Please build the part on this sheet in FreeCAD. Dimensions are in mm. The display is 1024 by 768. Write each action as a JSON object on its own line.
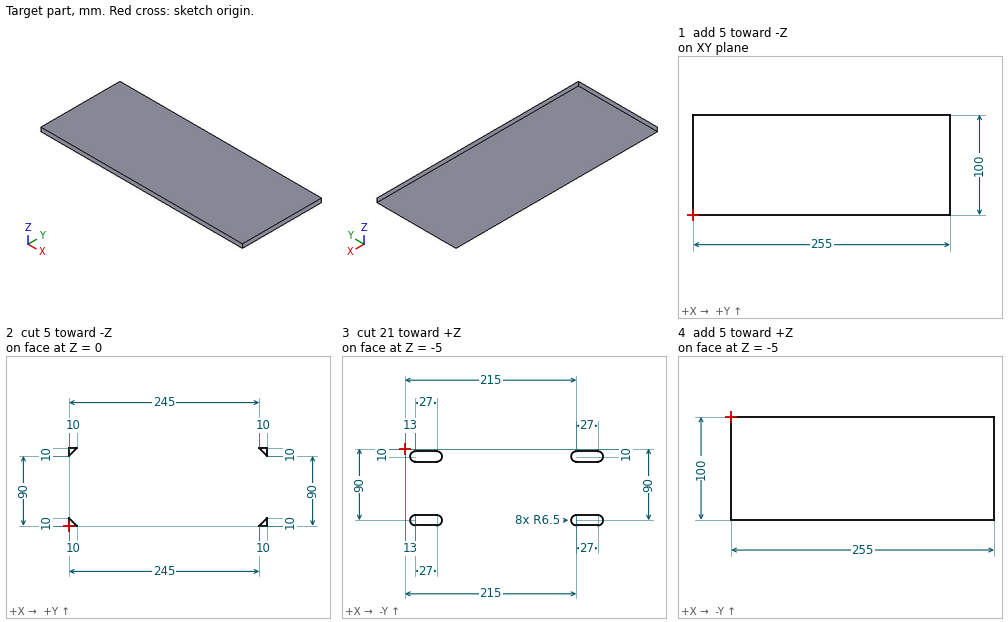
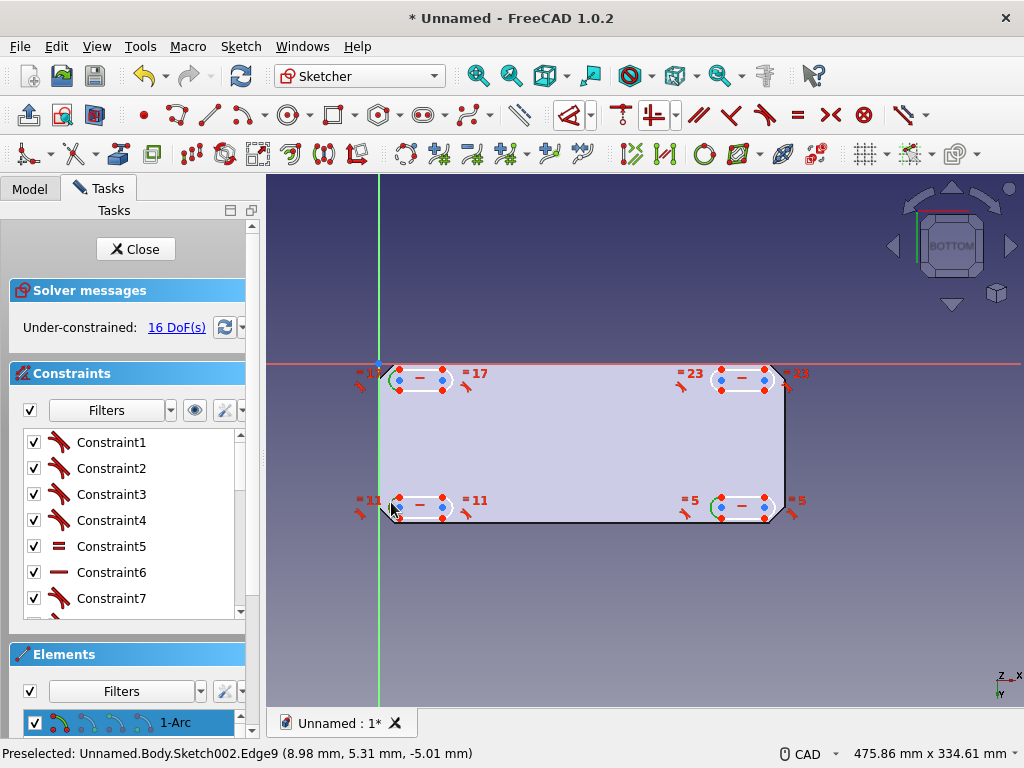
{"action": "scroll", "coordinate": [713, 374], "scroll_direction": "up", "scroll_amount": 2}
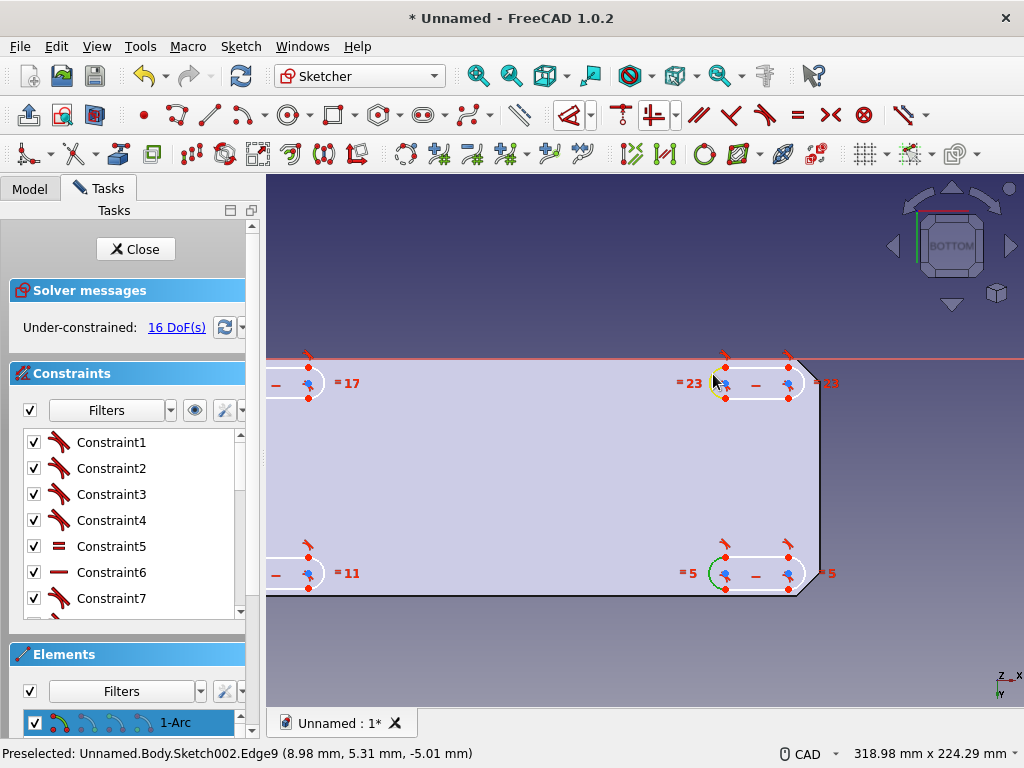
{"action": "left_click", "coordinate": [713, 374]}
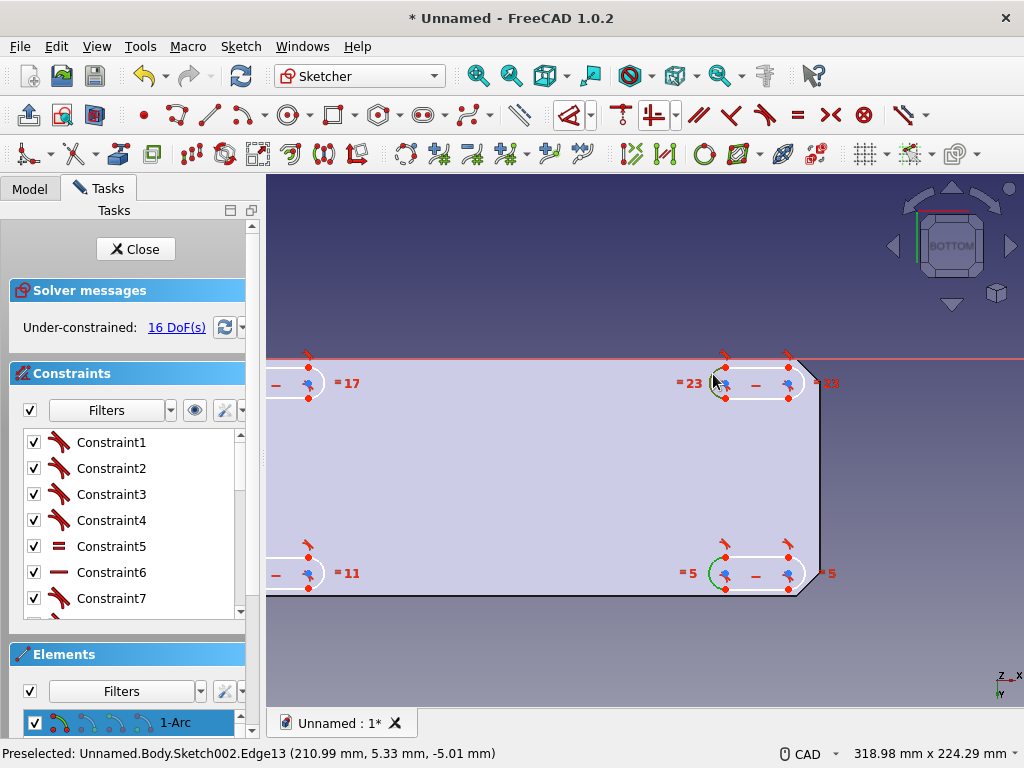
{"action": "key", "text": "e"}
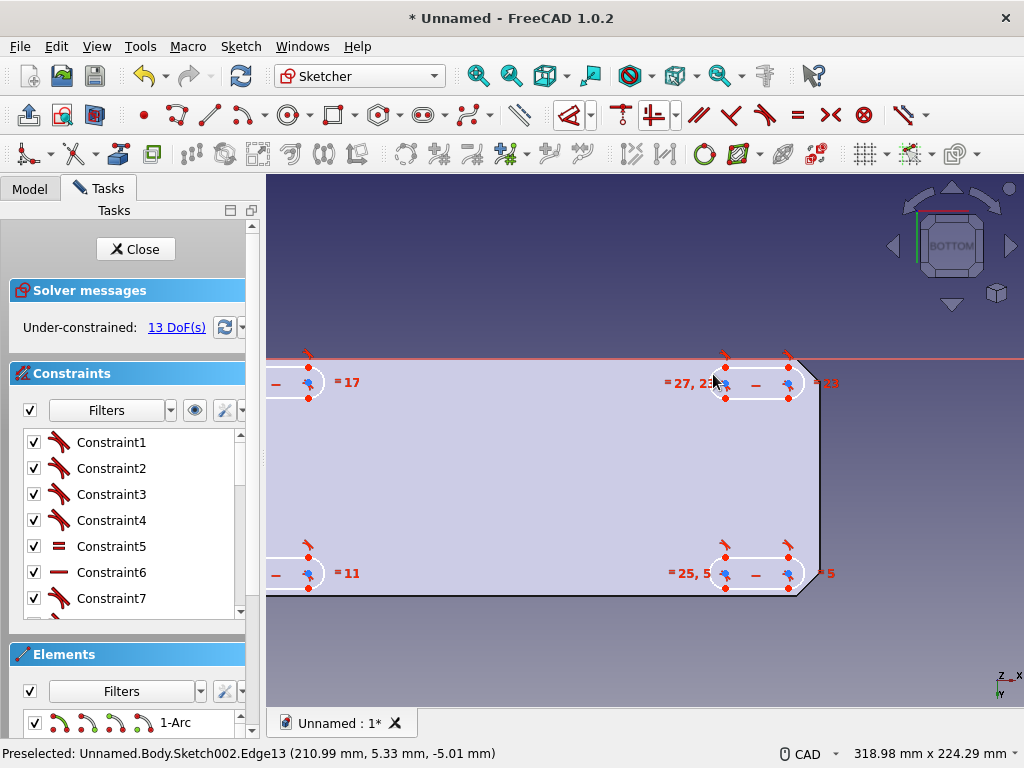
{"action": "key", "text": "d"}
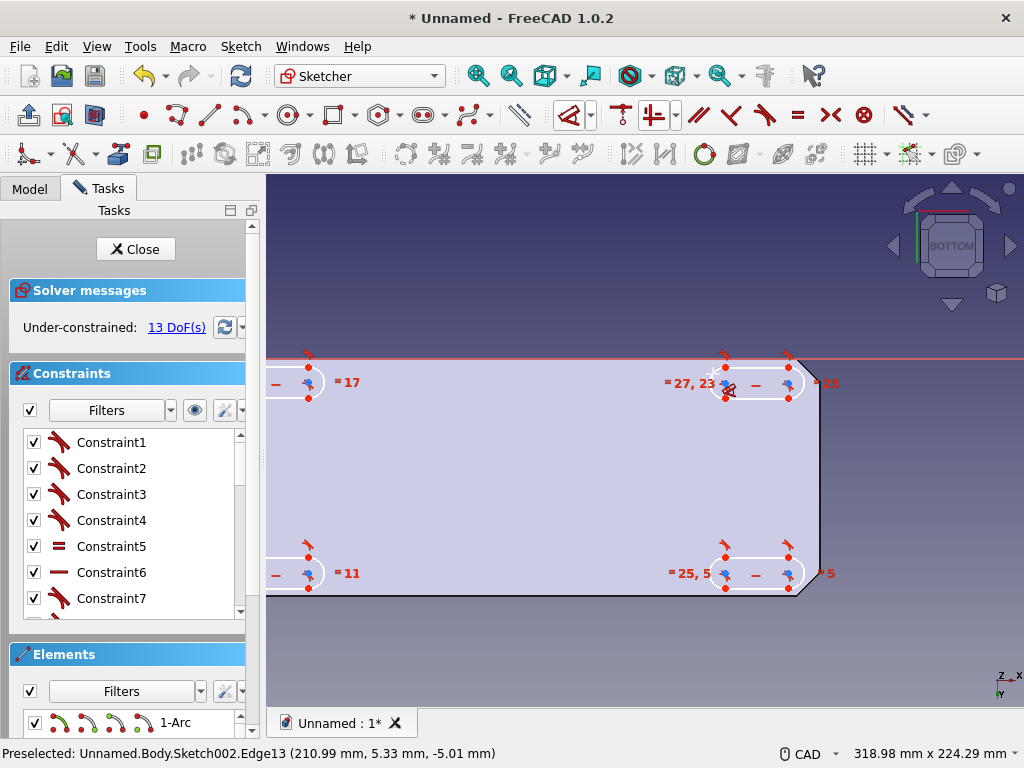
{"action": "scroll", "coordinate": [713, 564], "scroll_direction": "up", "scroll_amount": 5}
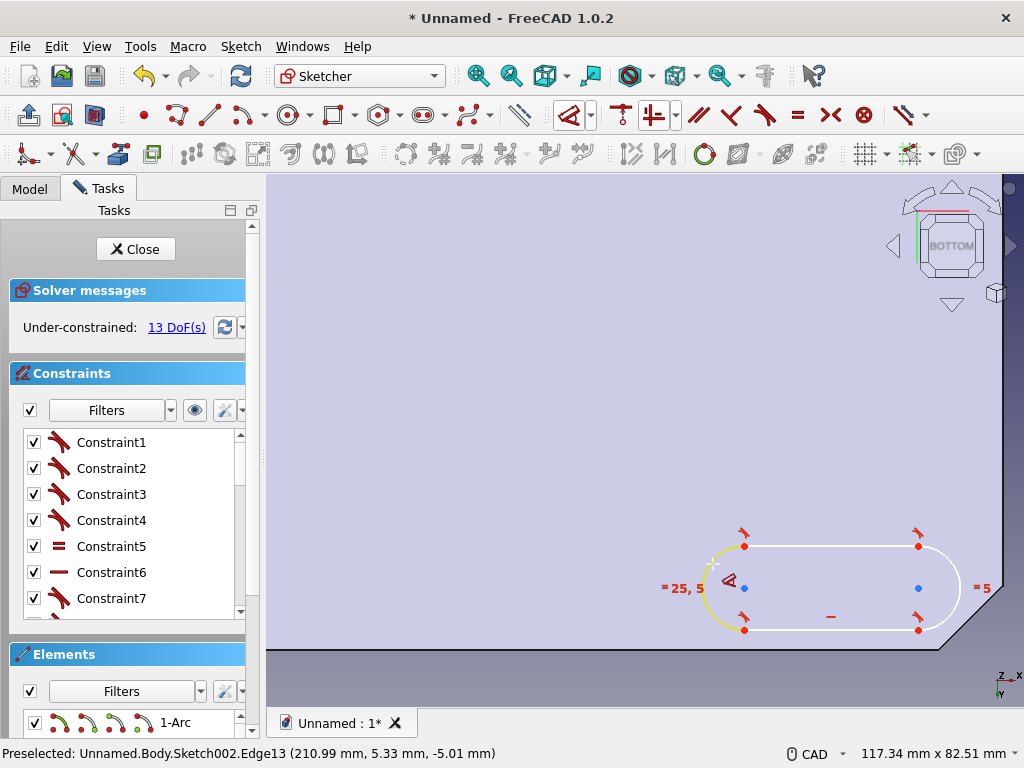
{"action": "left_click", "coordinate": [711, 563]}
{"action": "left_click", "coordinate": [685, 544]}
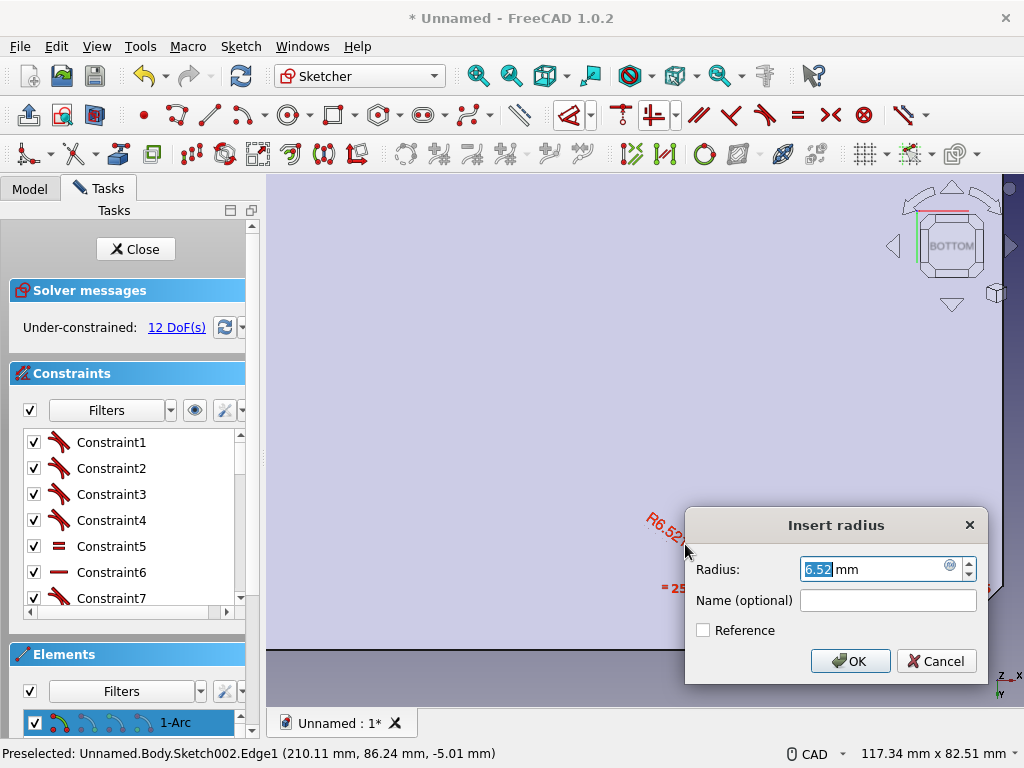
{"action": "type", "text": "6.5"}
{"action": "key", "text": "Return"}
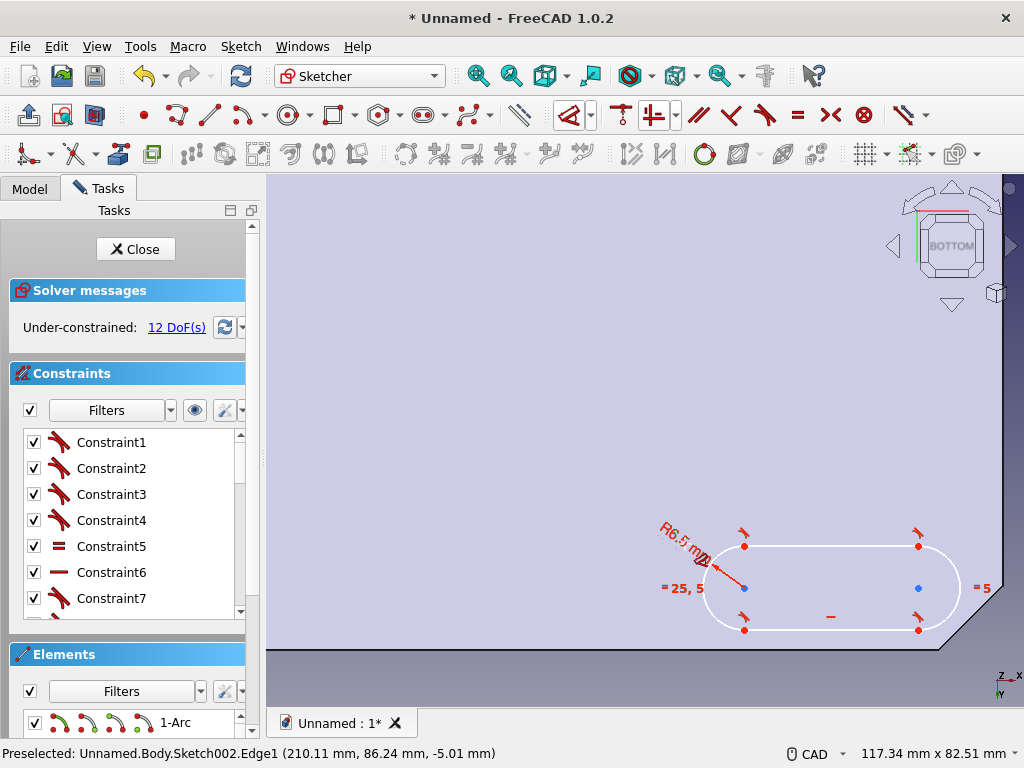
{"action": "scroll", "coordinate": [714, 481], "scroll_direction": "down", "scroll_amount": 7}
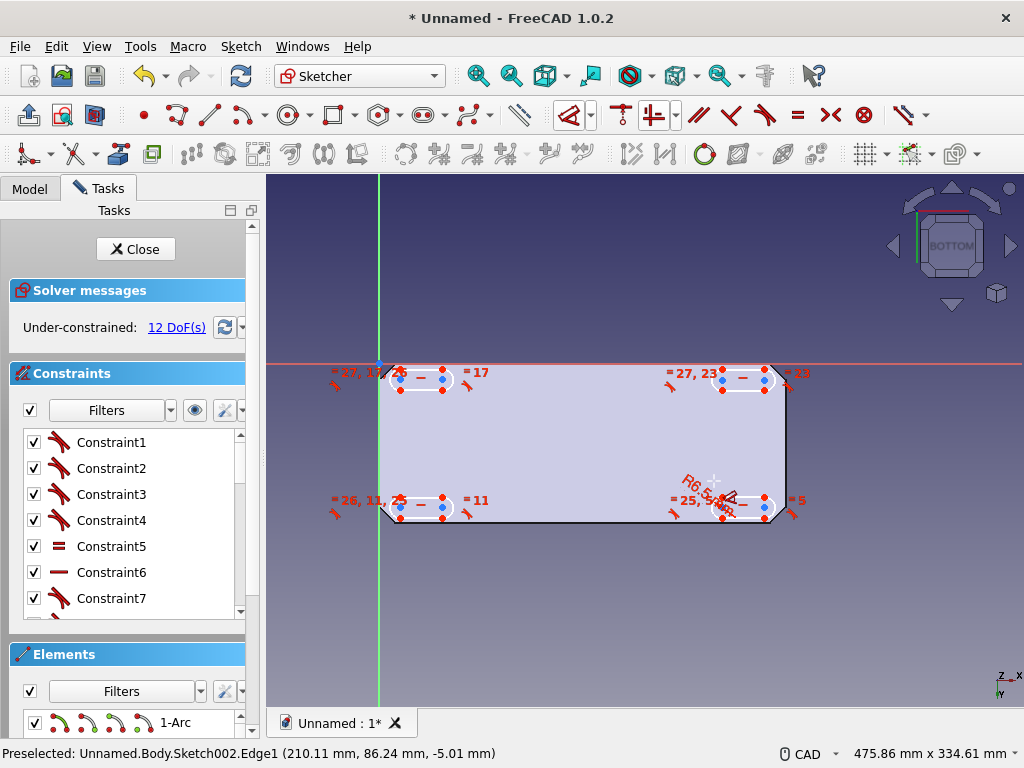
{"action": "left_click", "coordinate": [735, 497]}
{"action": "left_click", "coordinate": [743, 531]}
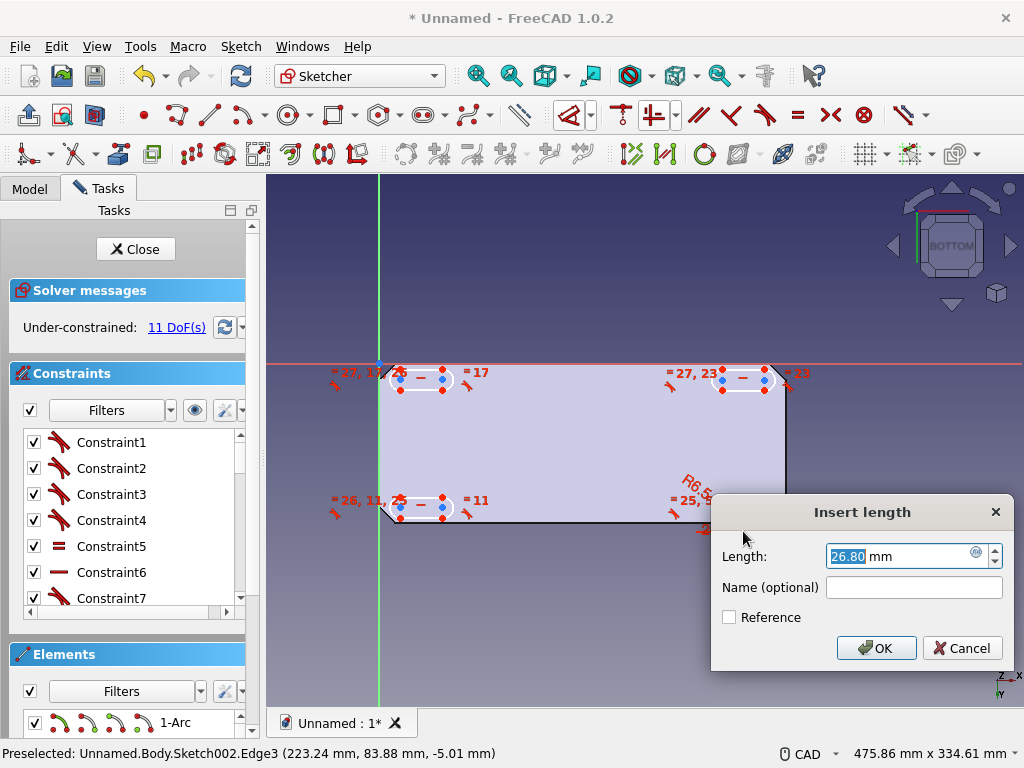
{"action": "type", "text": "27"}
{"action": "key", "text": "Return"}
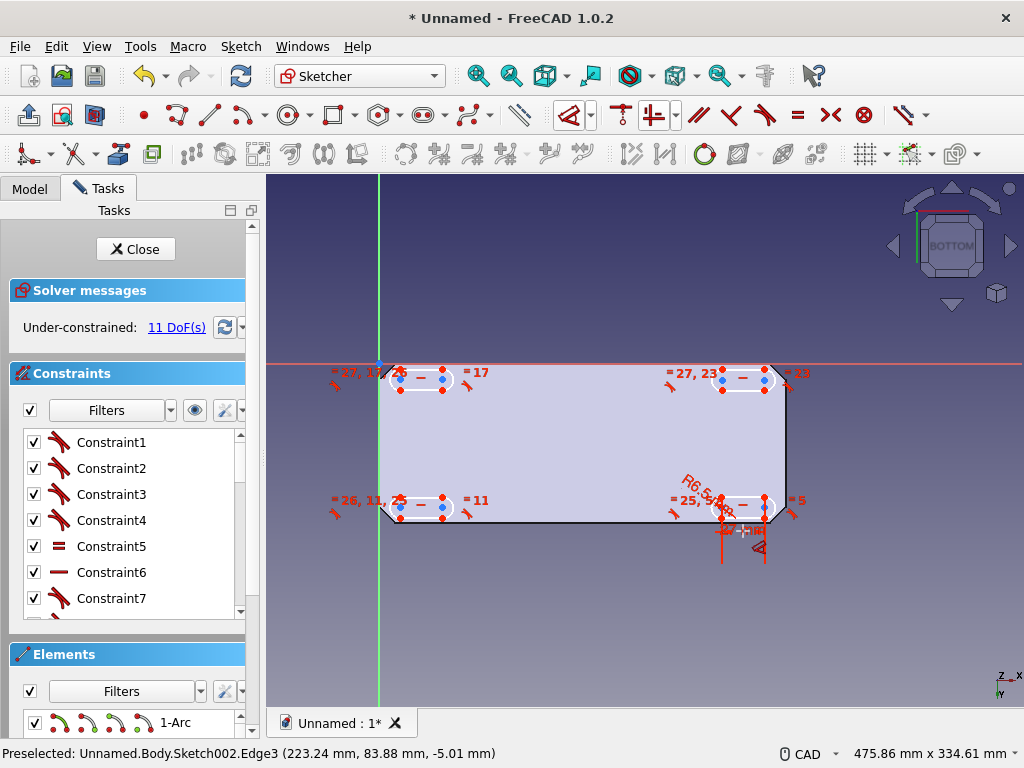
{"action": "left_click", "coordinate": [413, 498]}
{"action": "left_click", "coordinate": [422, 532]}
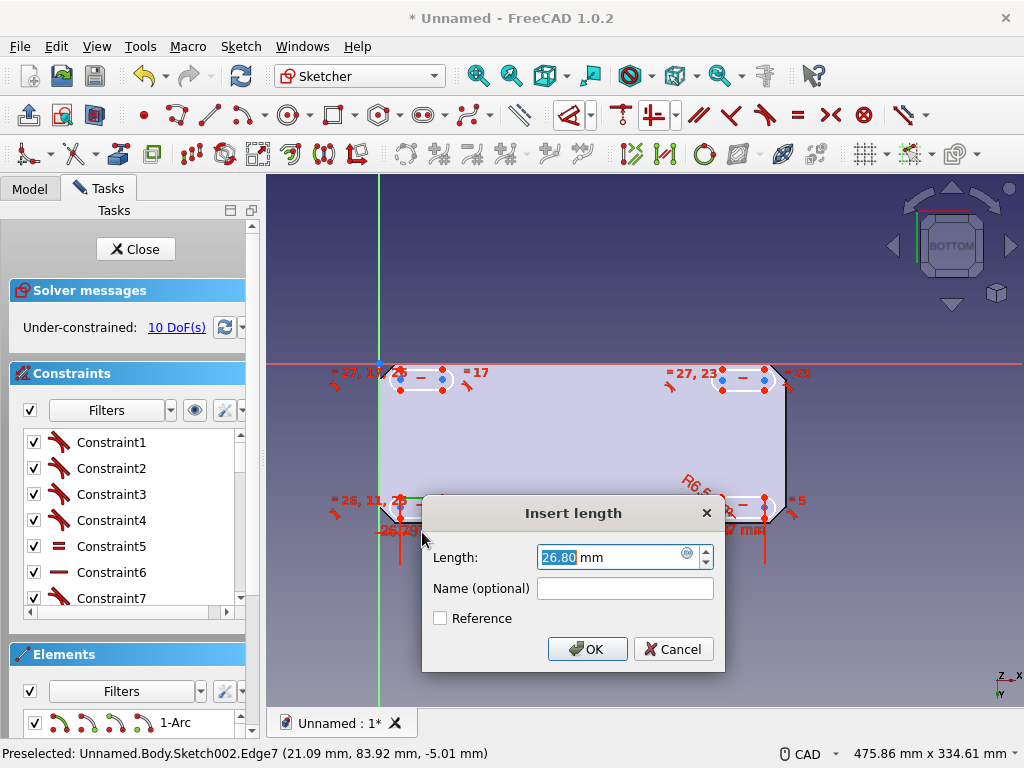
{"action": "type", "text": "27"}
{"action": "key", "text": "Return"}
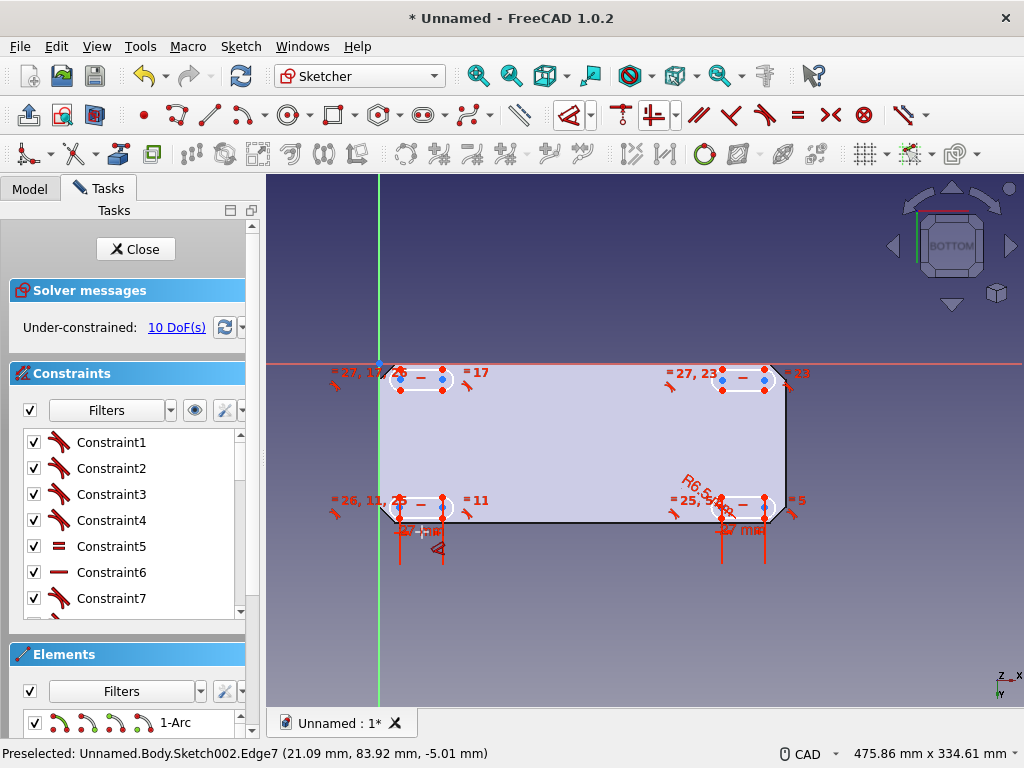
{"action": "scroll", "coordinate": [413, 370], "scroll_direction": "up", "scroll_amount": 5}